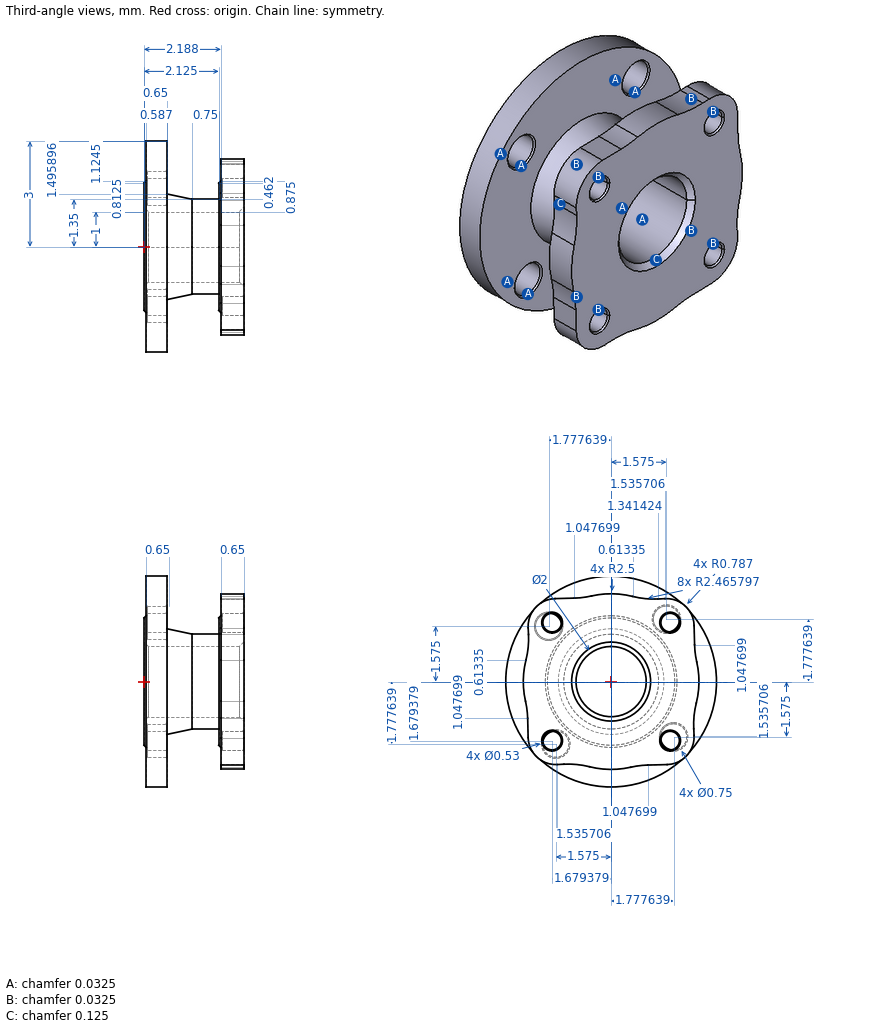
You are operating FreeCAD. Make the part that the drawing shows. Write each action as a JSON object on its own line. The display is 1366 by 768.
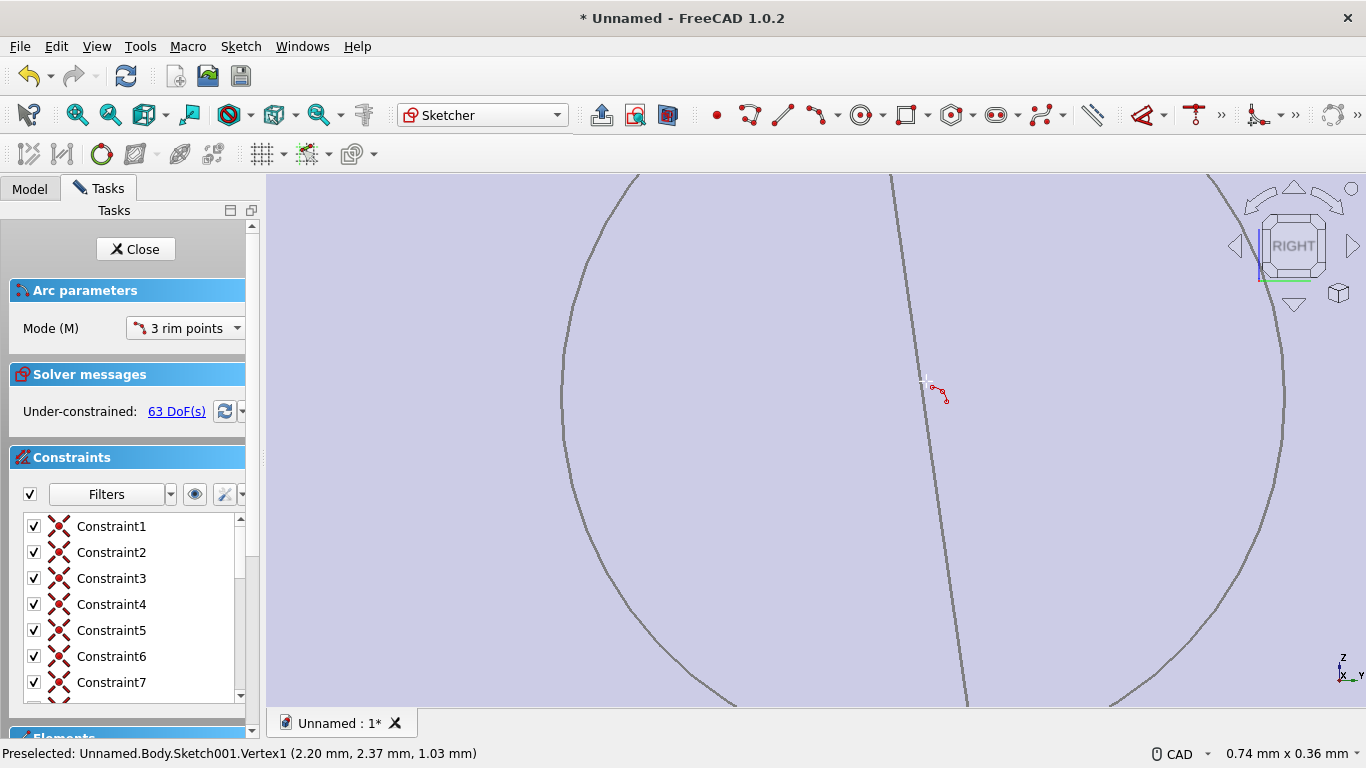
{"action": "left_click", "coordinate": [911, 377]}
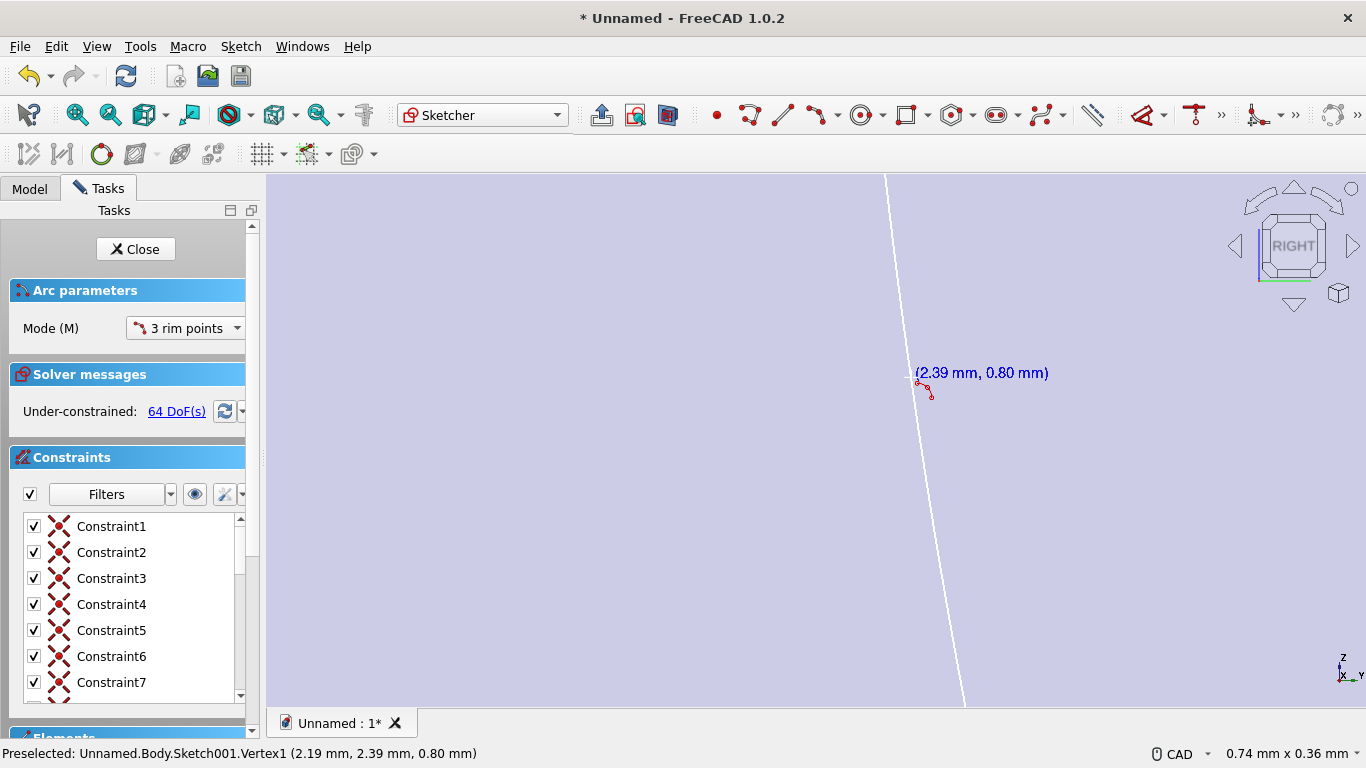
{"action": "left_click", "coordinate": [860, 116]}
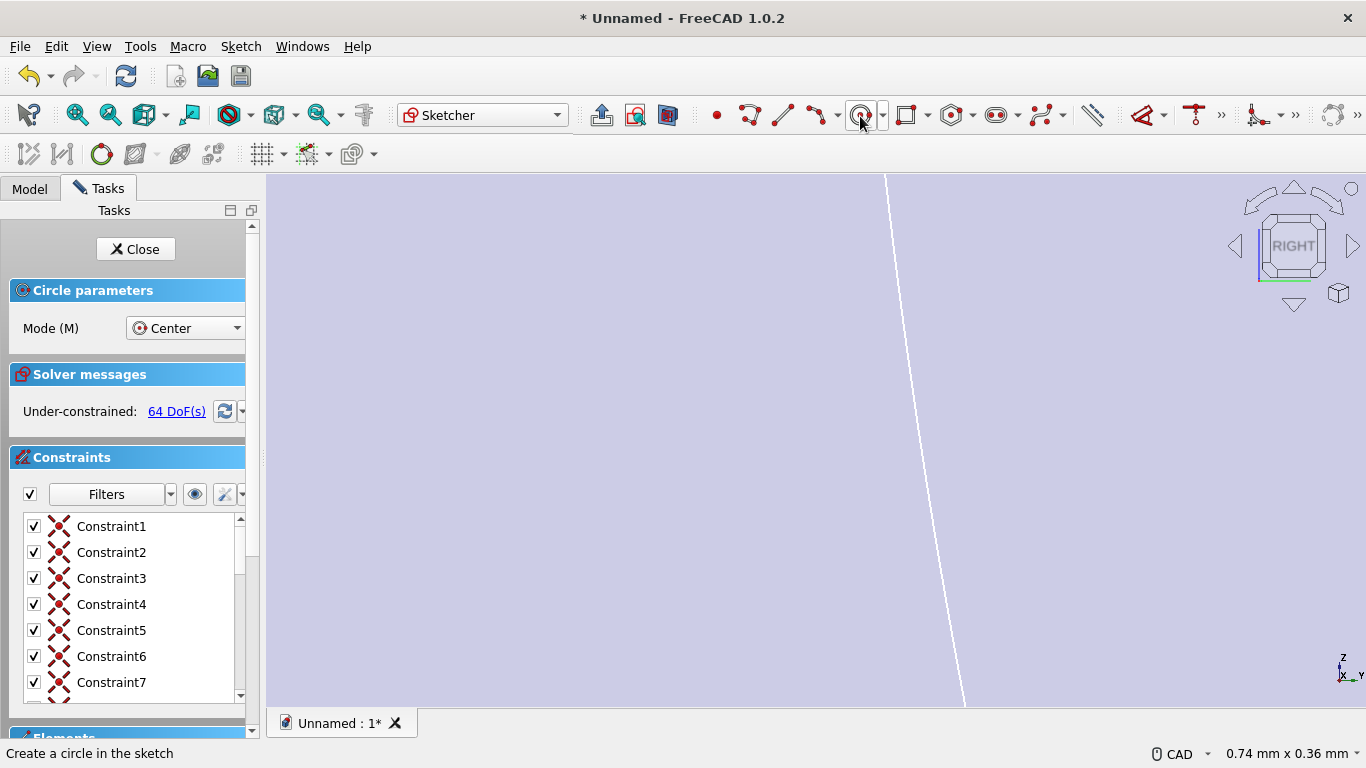
{"action": "scroll", "coordinate": [926, 381], "scroll_direction": "down", "scroll_amount": 15}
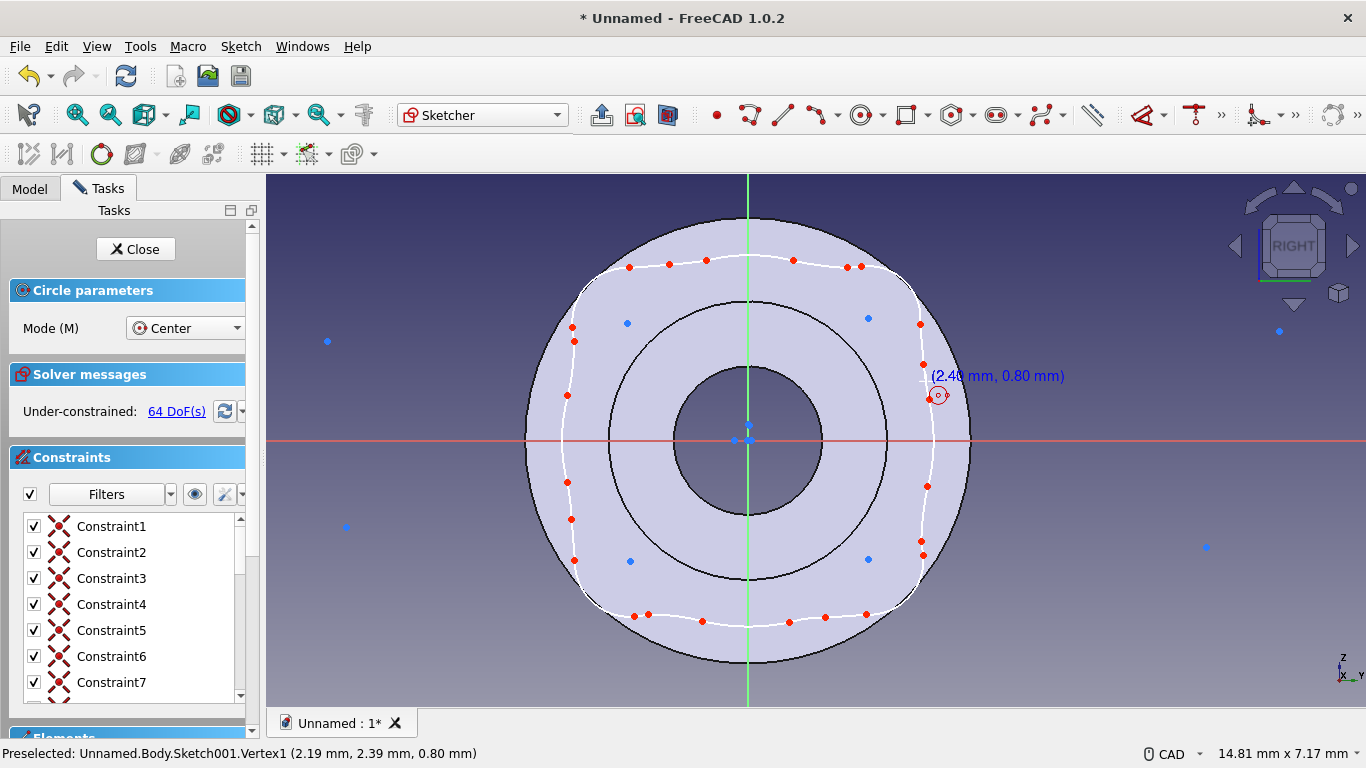
{"action": "scroll", "coordinate": [623, 565], "scroll_direction": "up", "scroll_amount": 2}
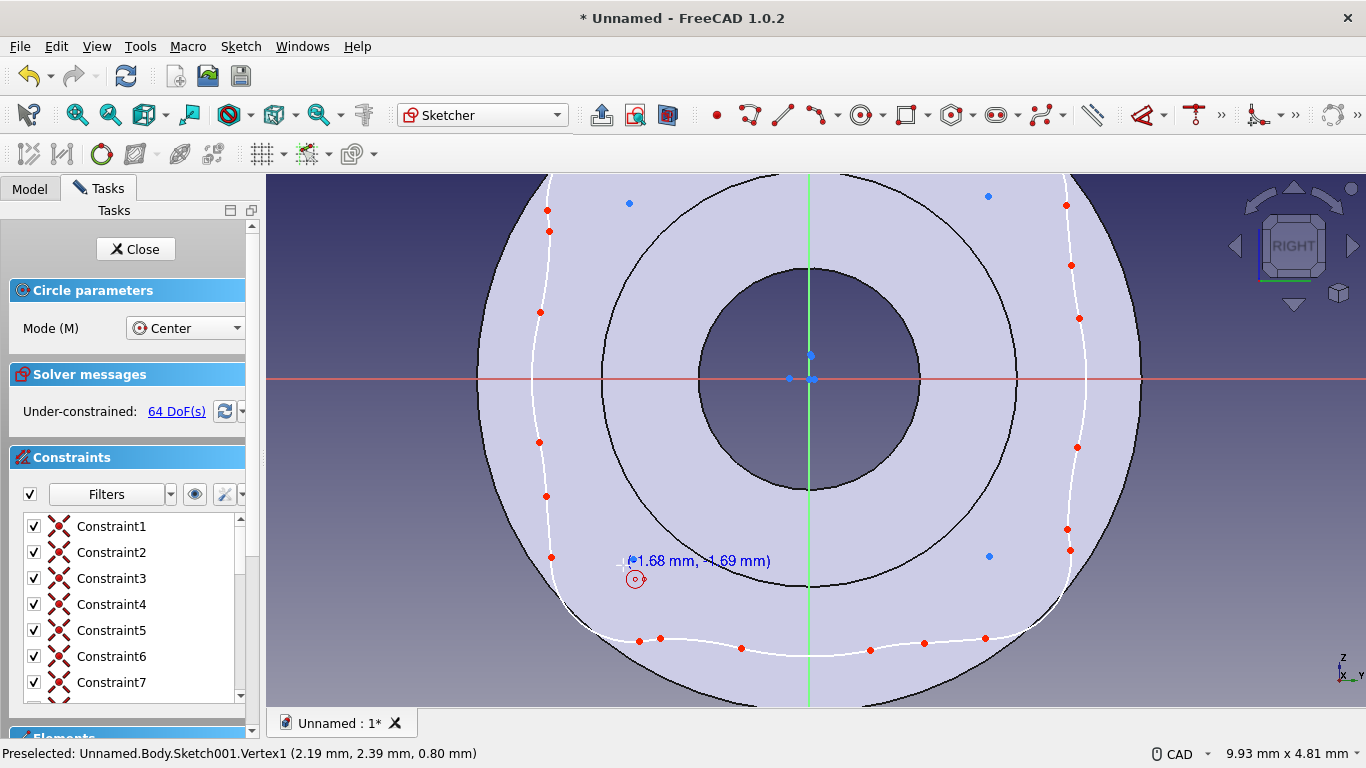
{"action": "left_click", "coordinate": [623, 565]}
{"action": "left_click", "coordinate": [602, 545]}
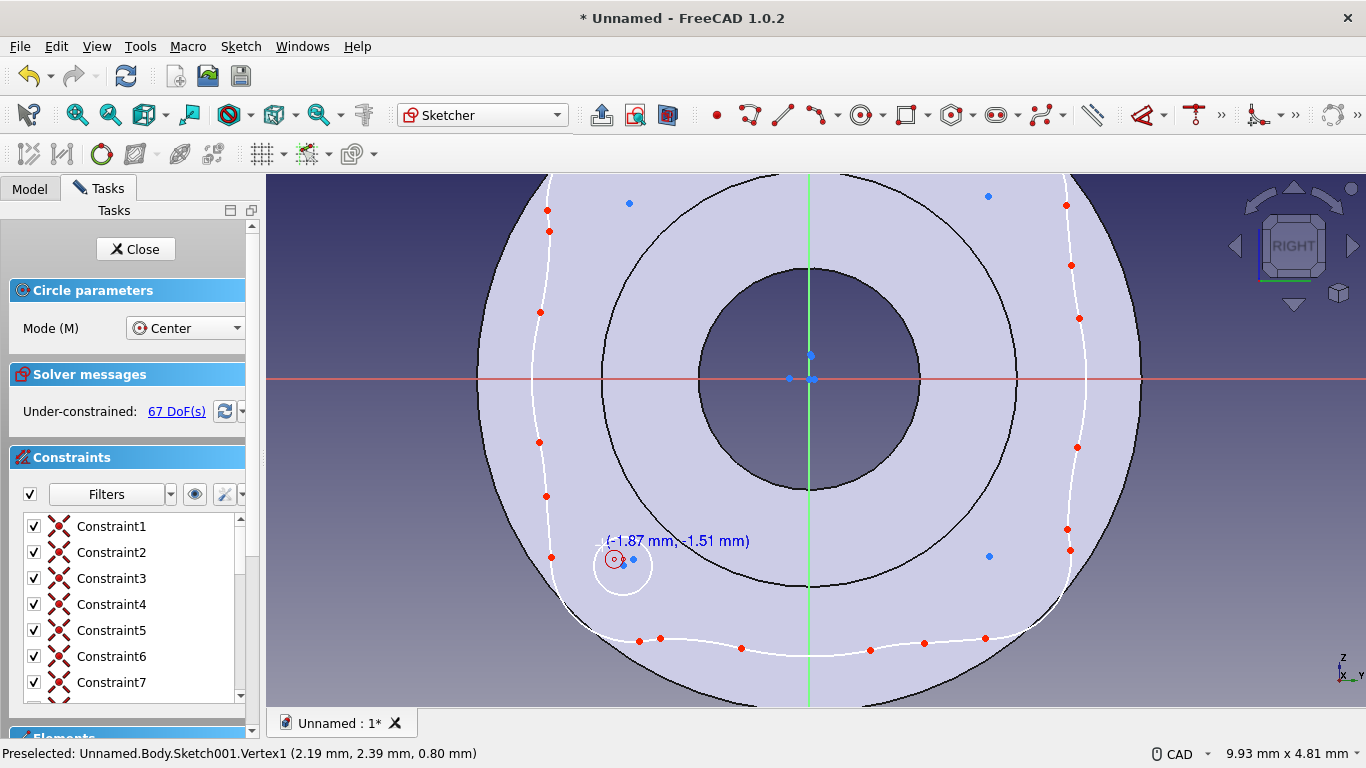
{"action": "scroll", "coordinate": [622, 565], "scroll_direction": "down", "scroll_amount": 2}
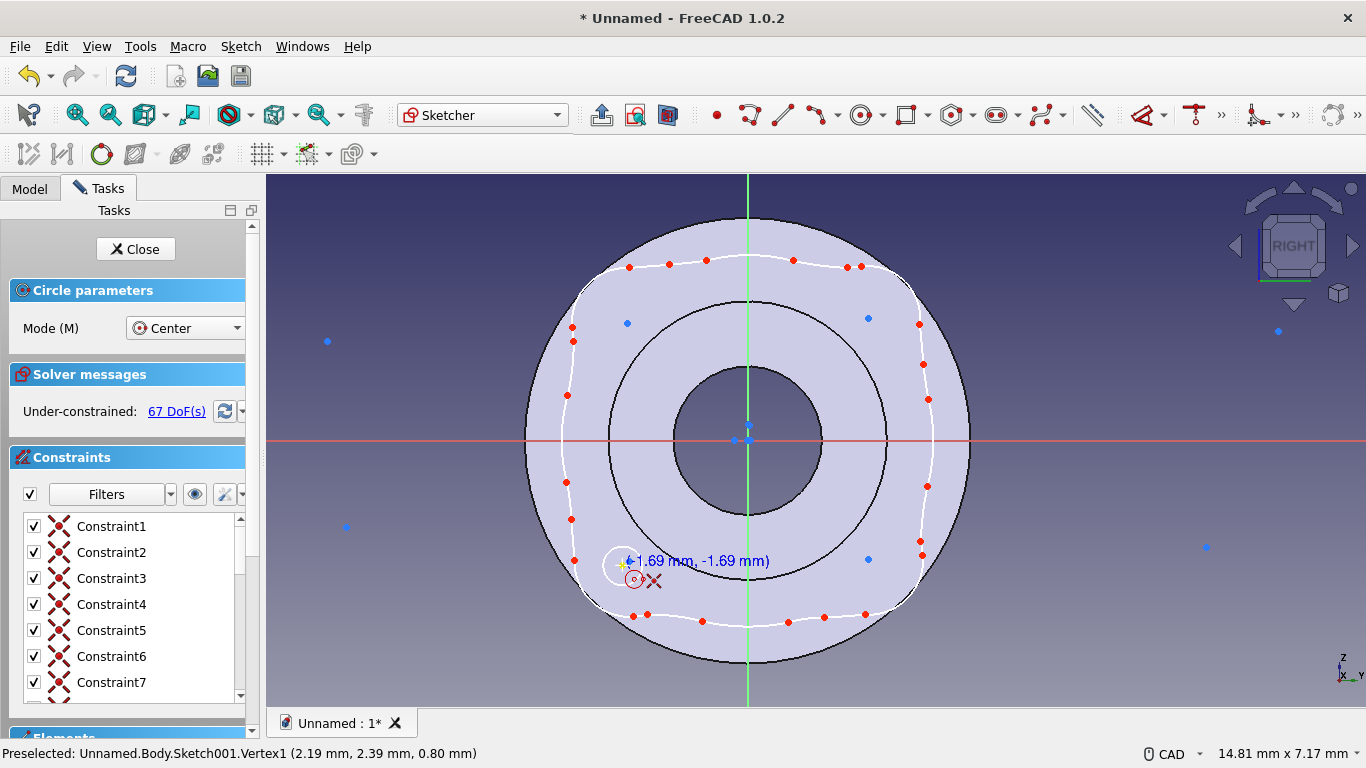
{"action": "scroll", "coordinate": [623, 316], "scroll_direction": "up", "scroll_amount": 2}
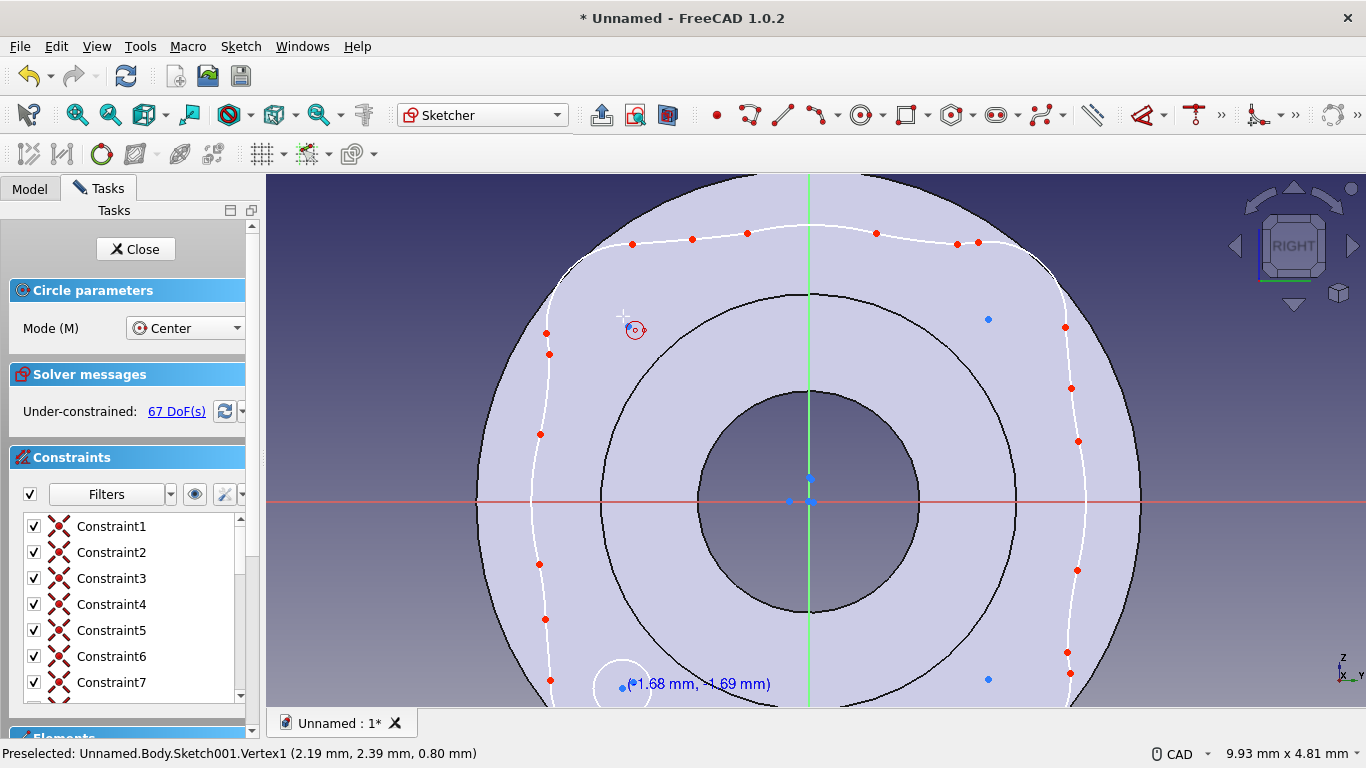
{"action": "left_click", "coordinate": [623, 316]}
{"action": "left_click", "coordinate": [643, 295]}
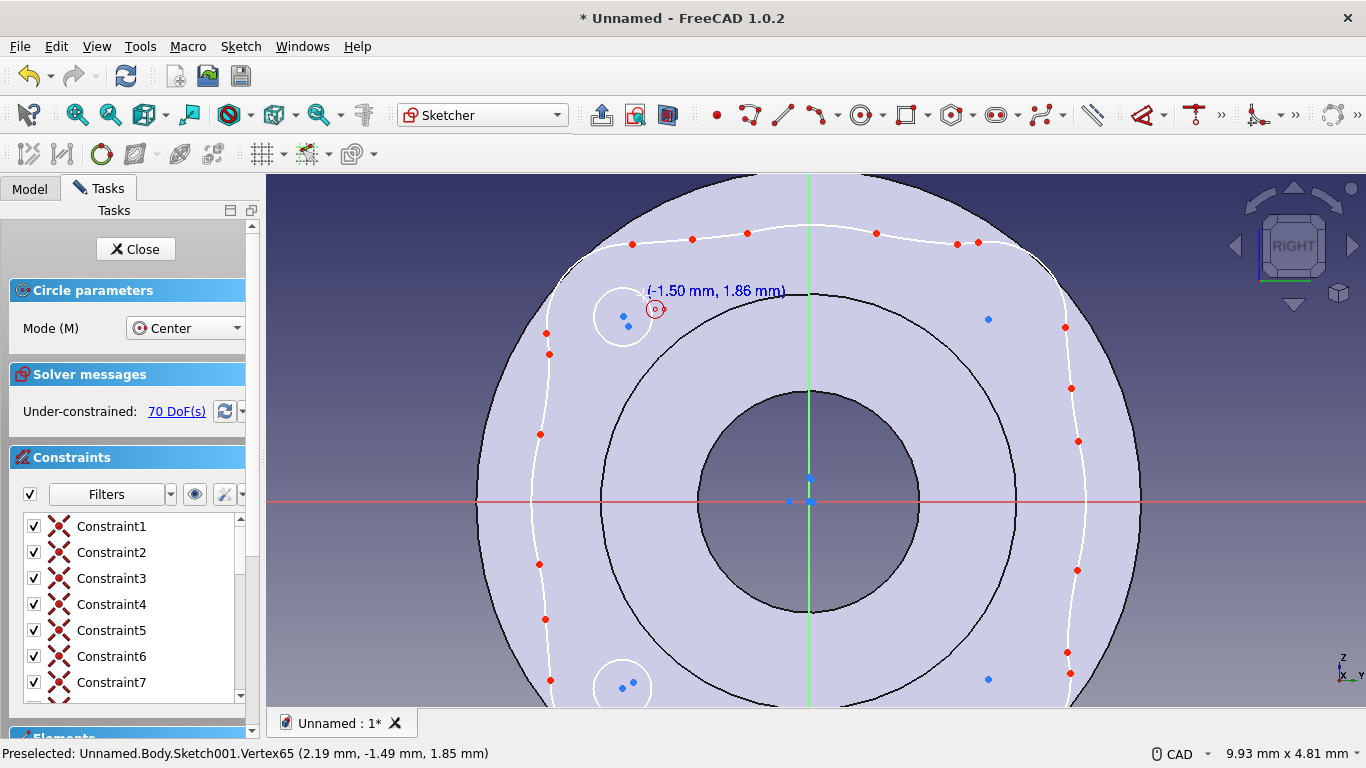
{"action": "scroll", "coordinate": [623, 316], "scroll_direction": "down", "scroll_amount": 2}